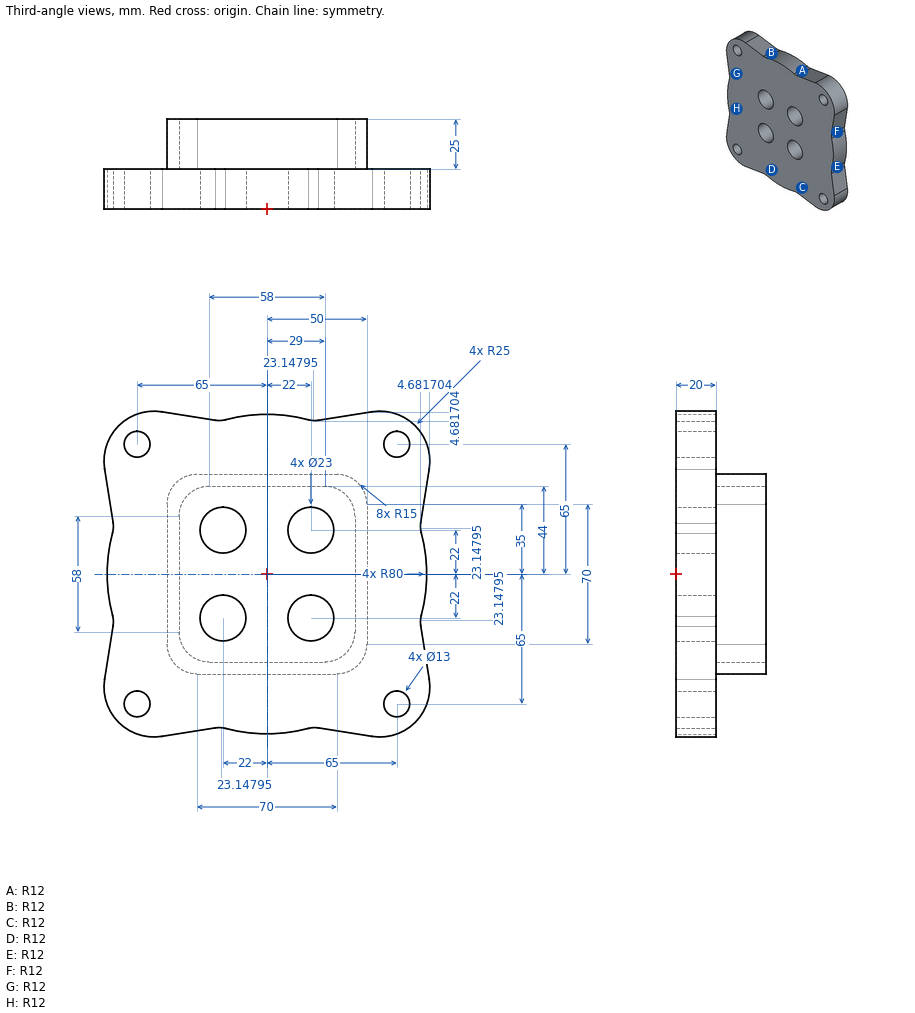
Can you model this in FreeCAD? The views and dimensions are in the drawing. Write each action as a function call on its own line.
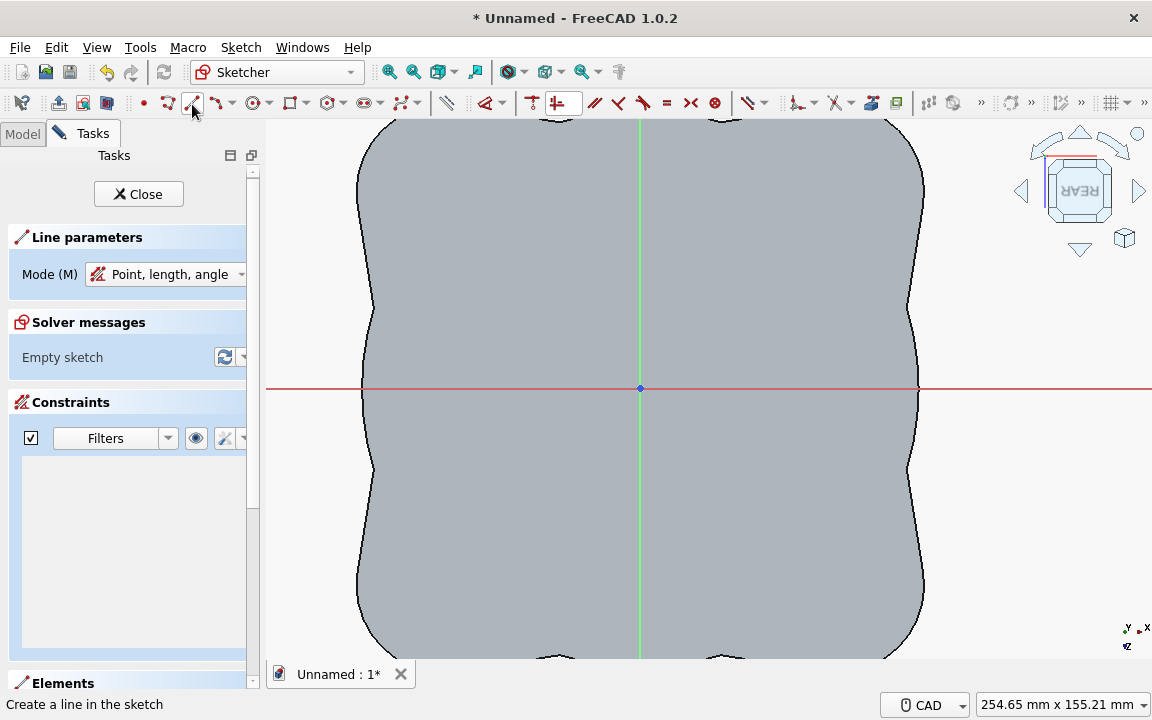
click(814, 511)
click(814, 267)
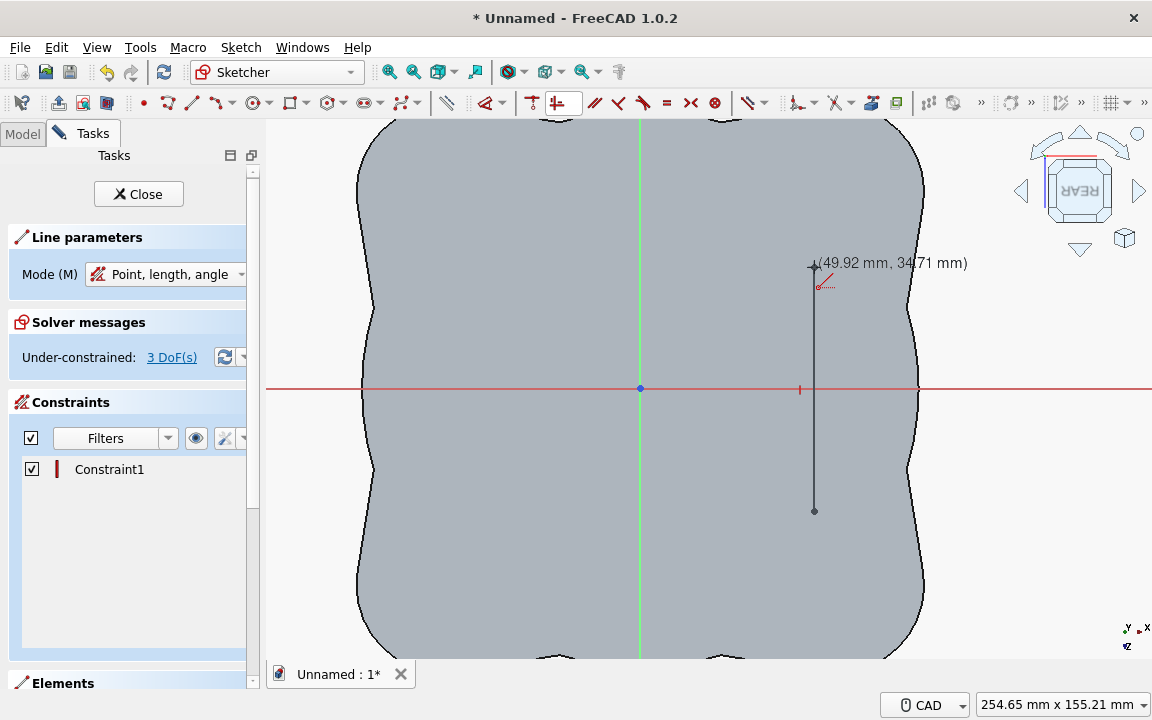
click(762, 215)
click(519, 215)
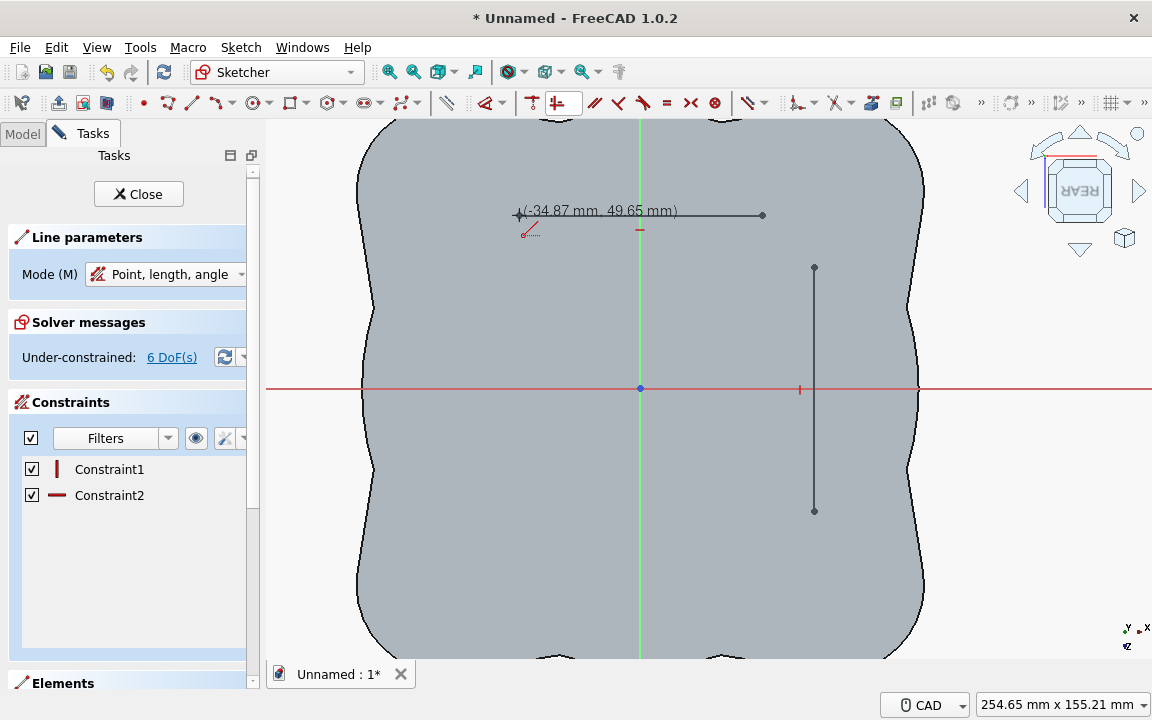
click(466, 267)
click(466, 511)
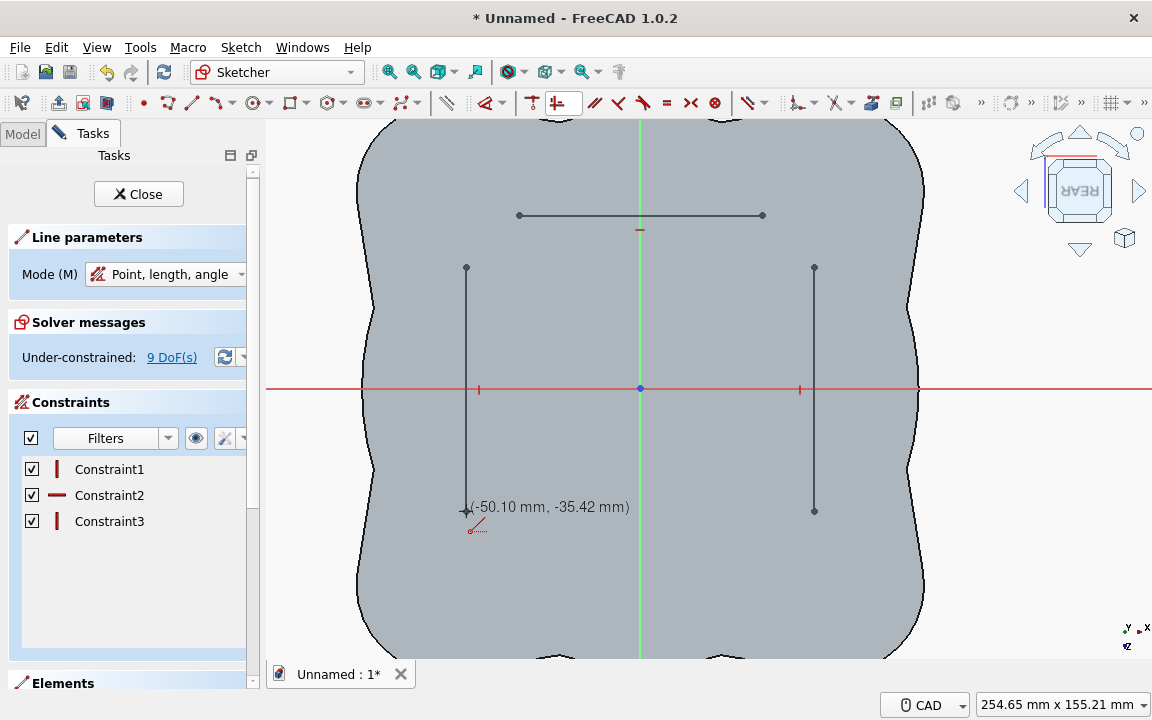
click(519, 563)
click(762, 563)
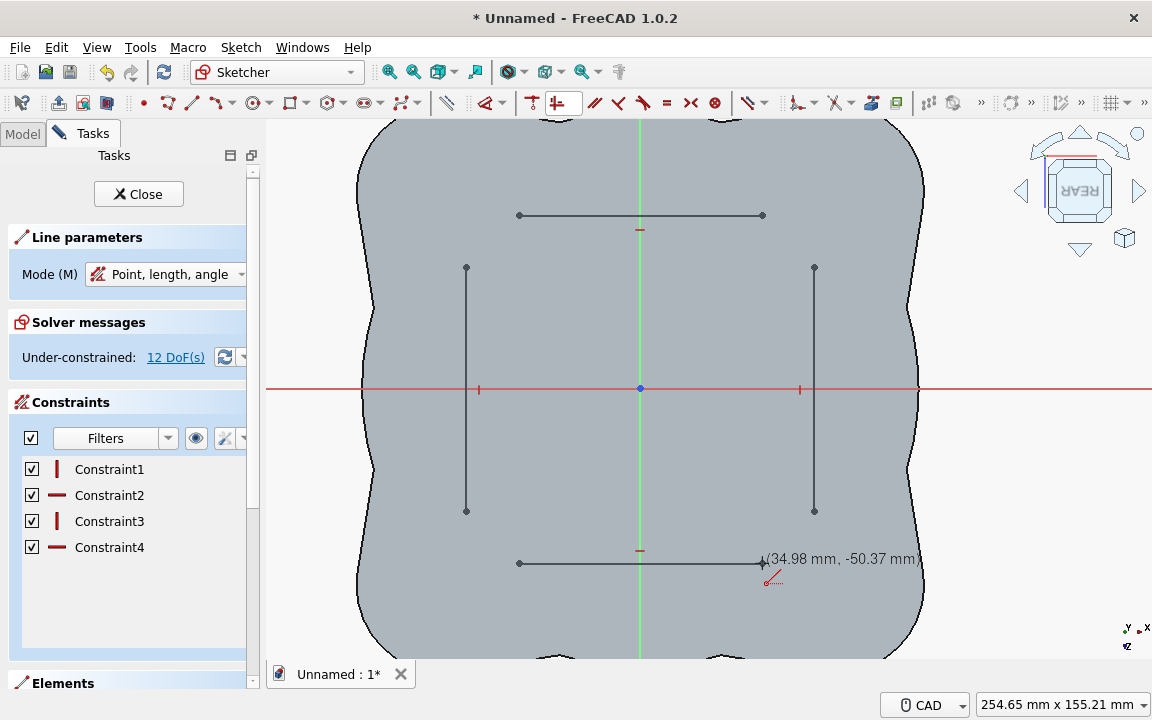
click(216, 104)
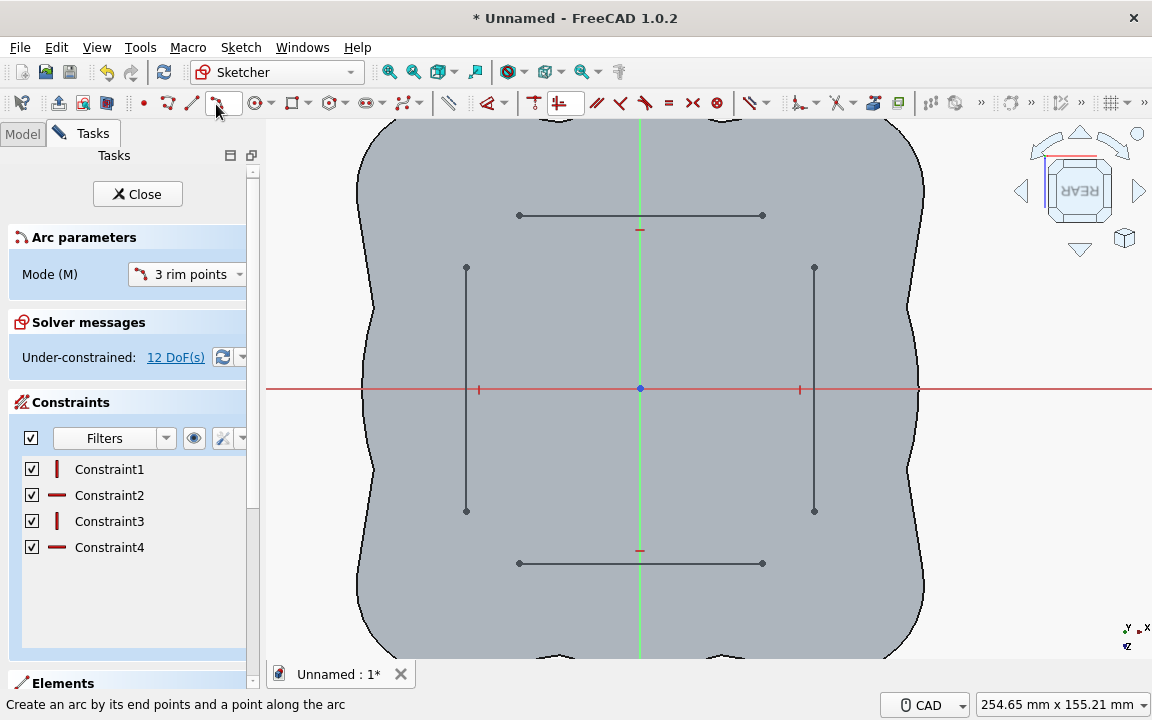
click(814, 268)
click(762, 216)
click(799, 230)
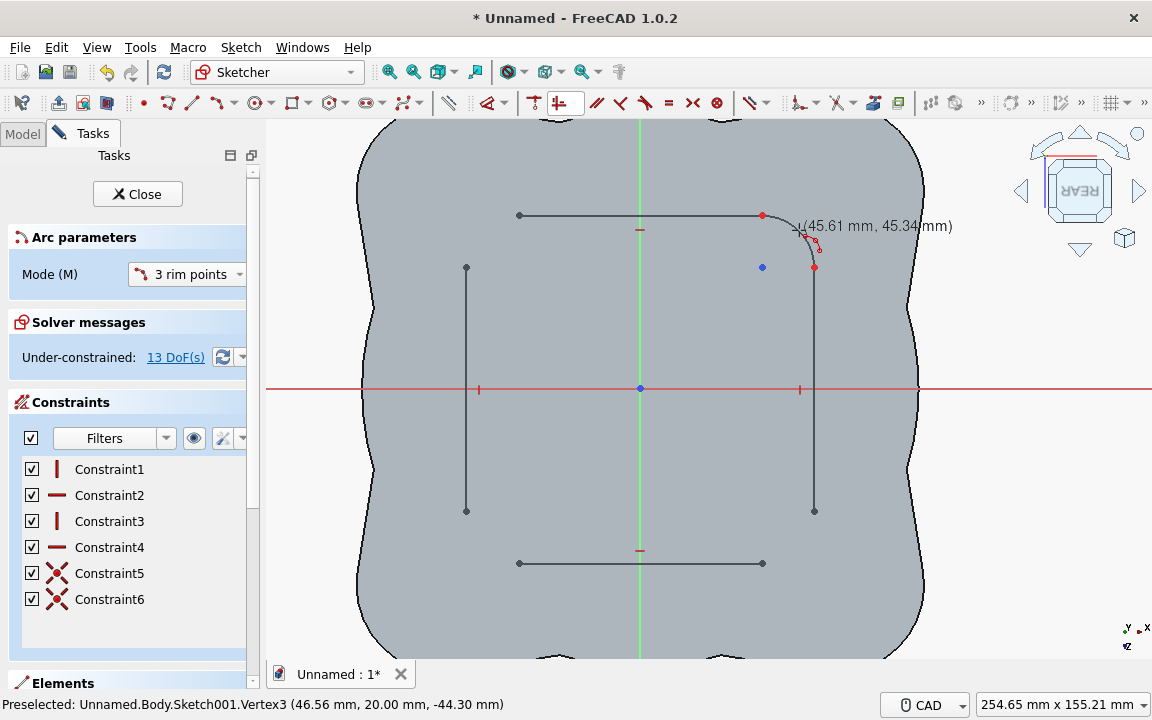
click(519, 216)
click(466, 268)
click(482, 230)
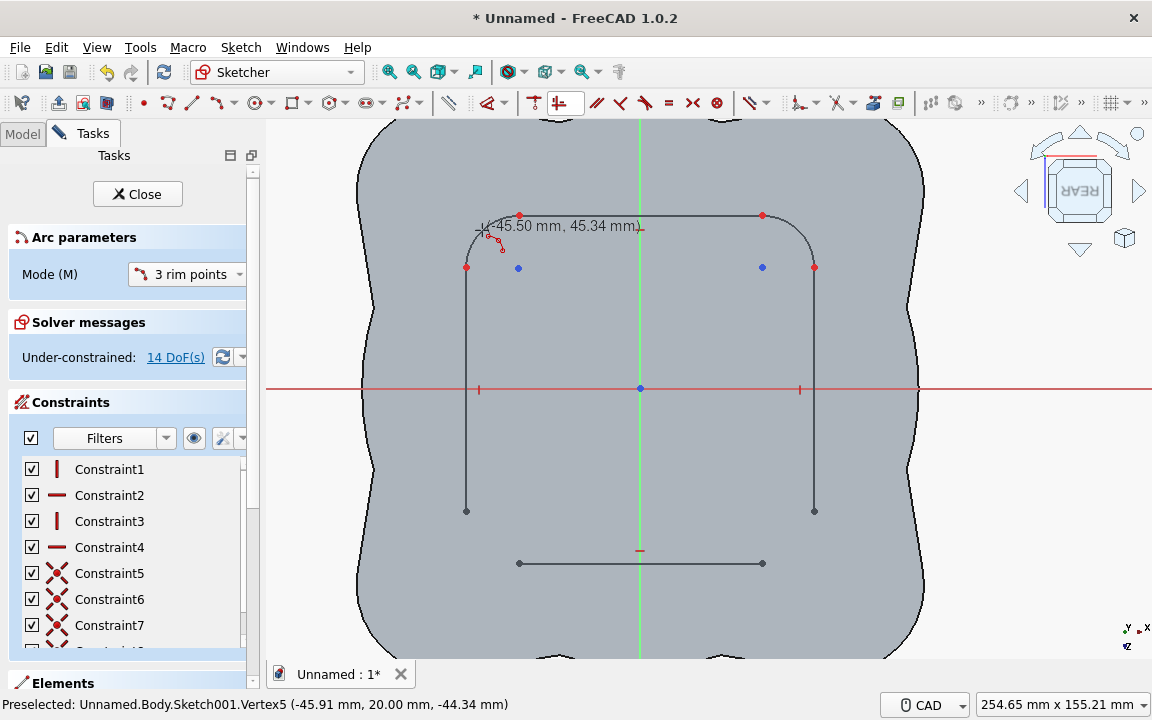
click(466, 512)
click(519, 564)
click(482, 547)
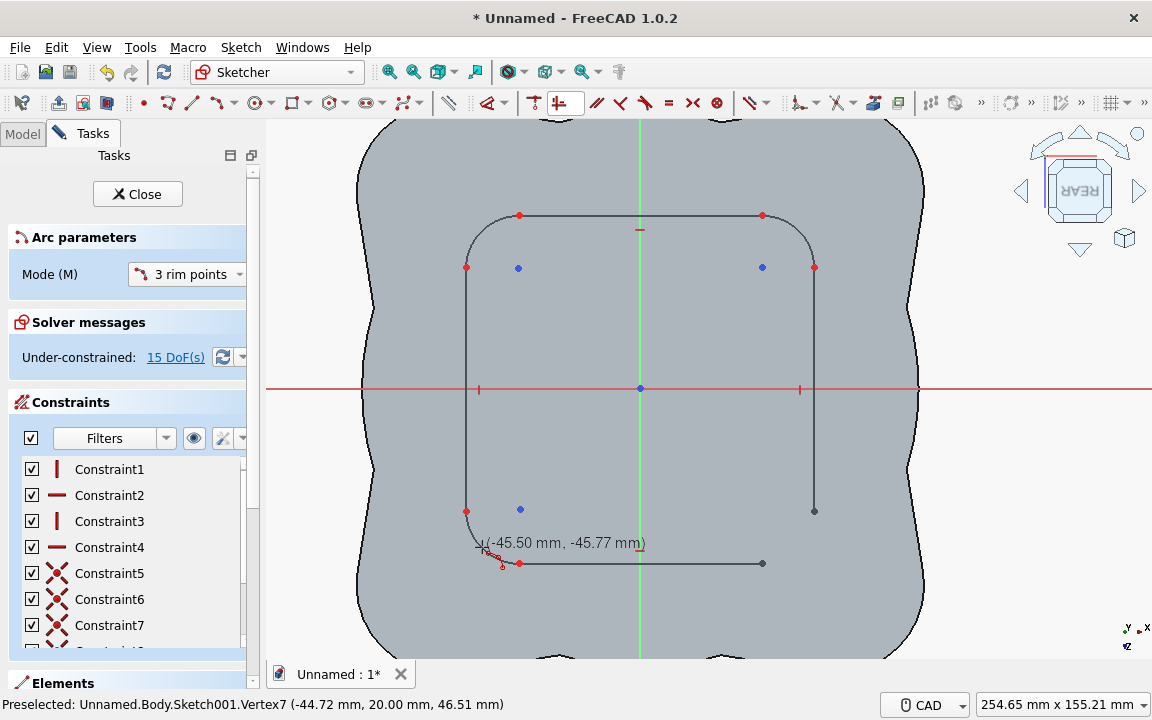
click(762, 564)
click(814, 512)
click(799, 547)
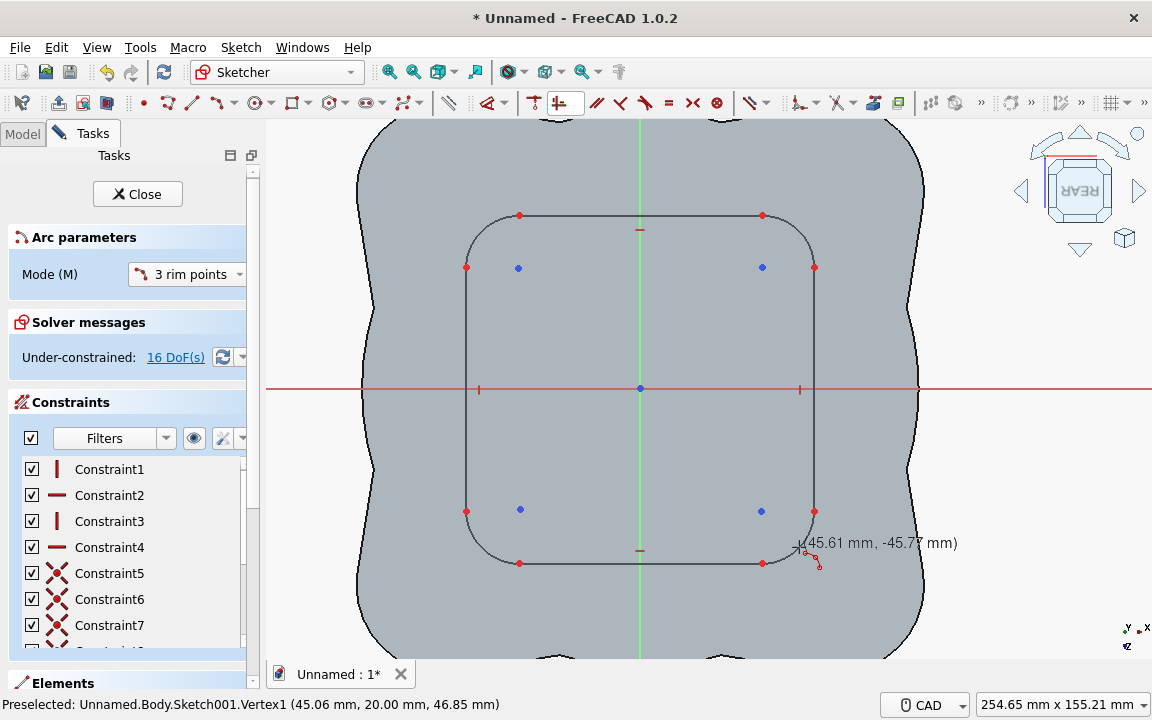
click(192, 104)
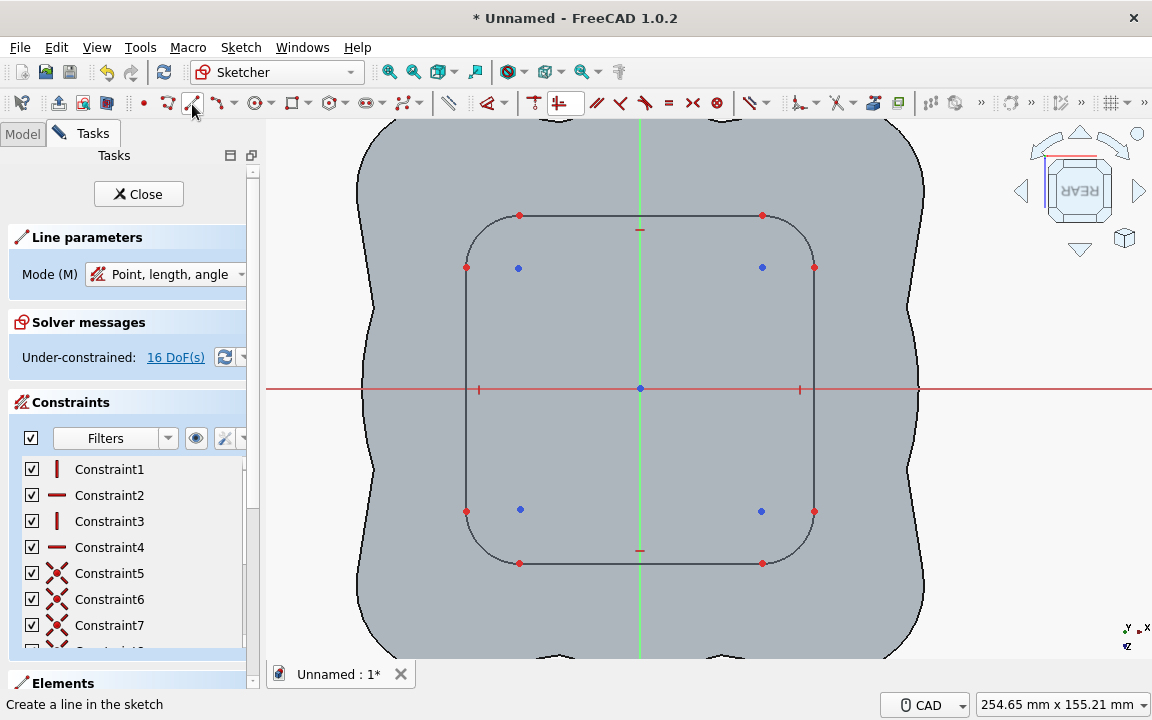
click(741, 542)
click(539, 542)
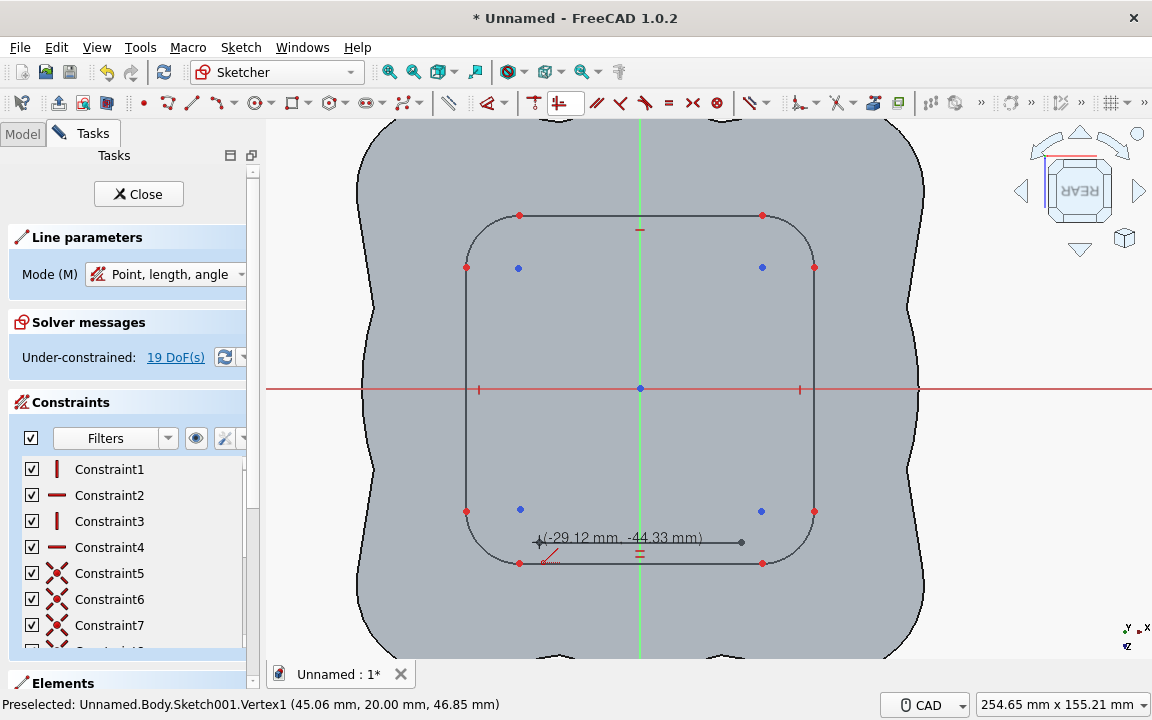
click(487, 490)
click(487, 288)